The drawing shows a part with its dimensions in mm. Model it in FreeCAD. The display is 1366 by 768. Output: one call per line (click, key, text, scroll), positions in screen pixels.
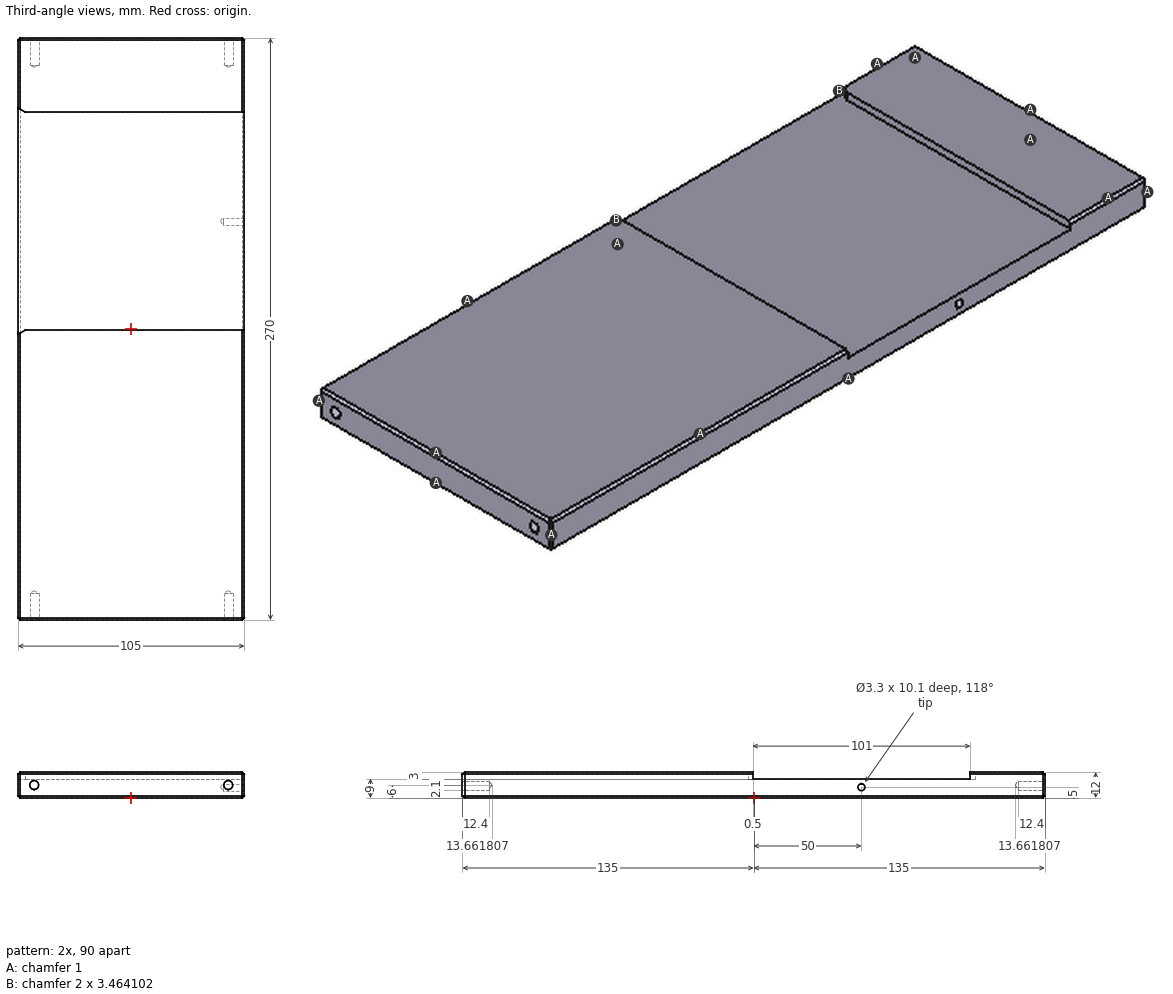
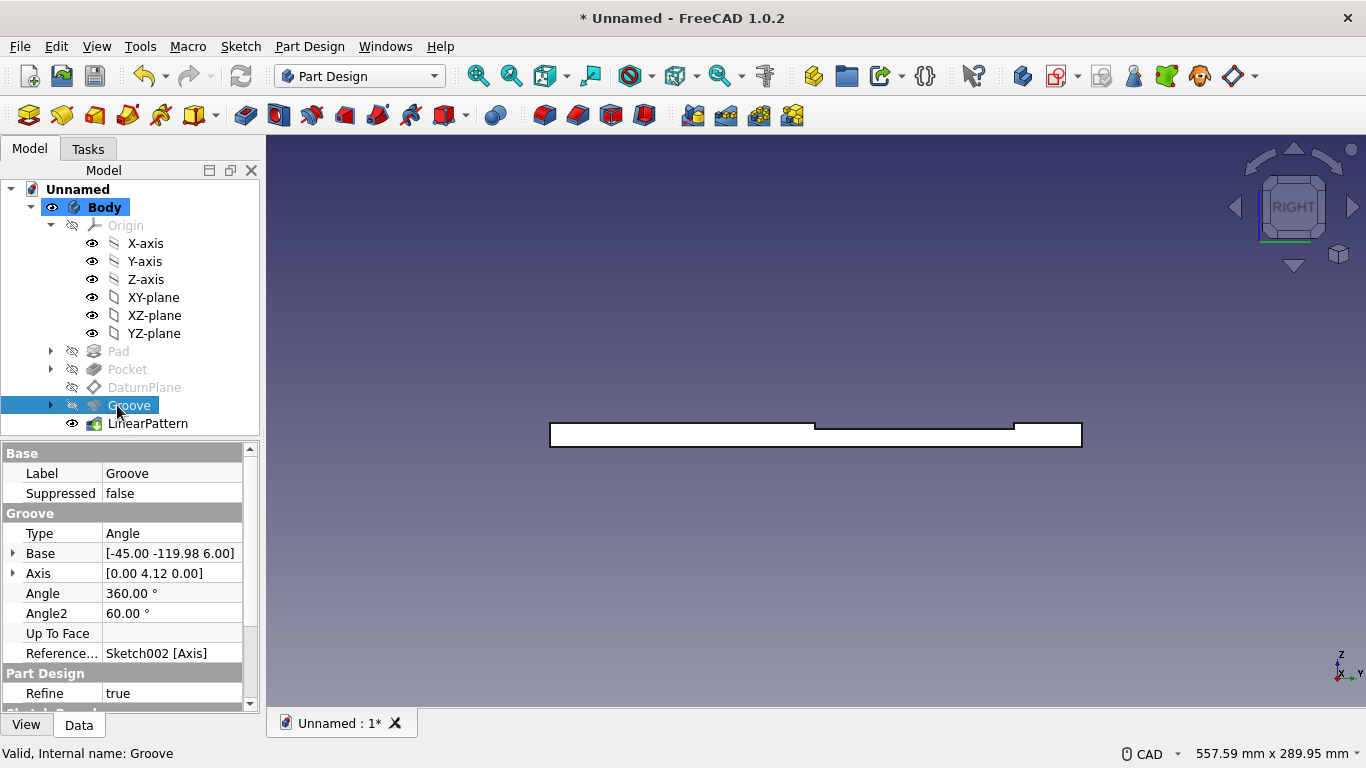
click(693, 116)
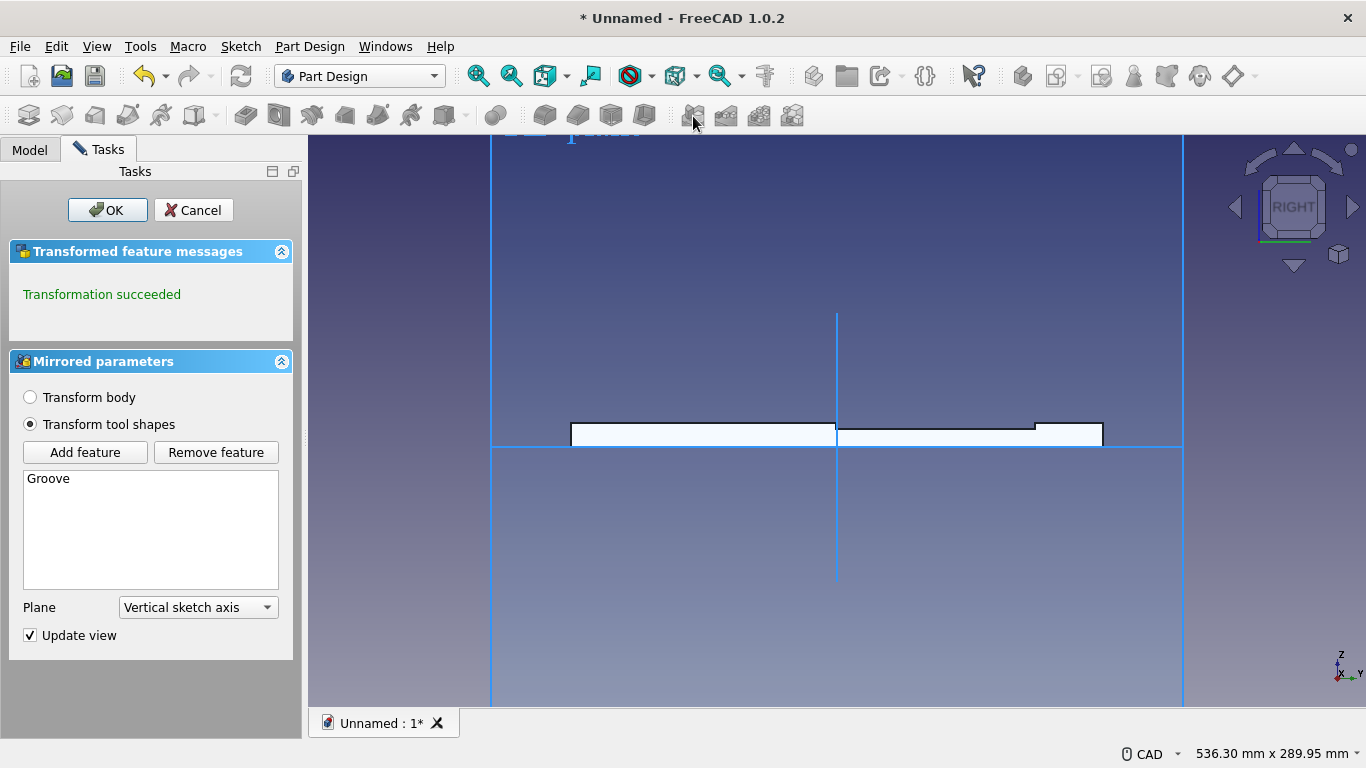
click(199, 608)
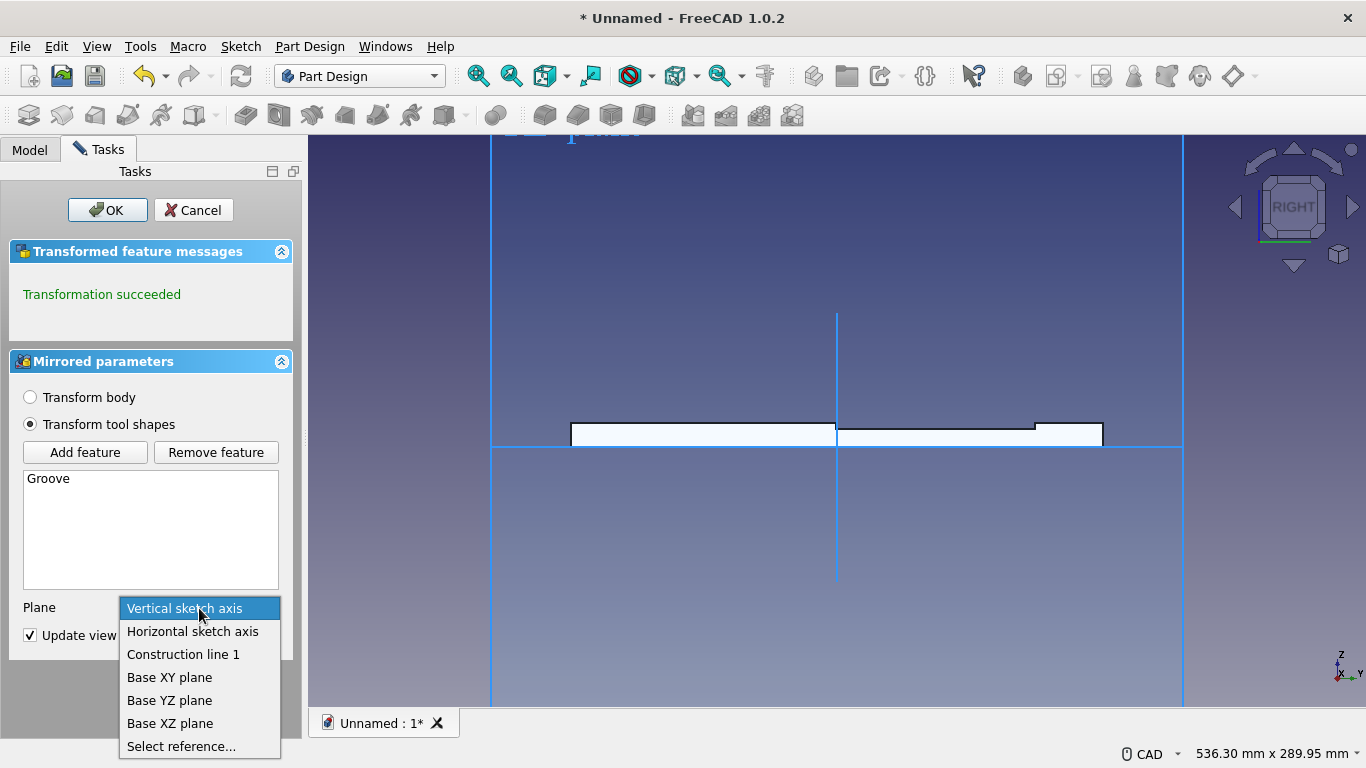
click(198, 724)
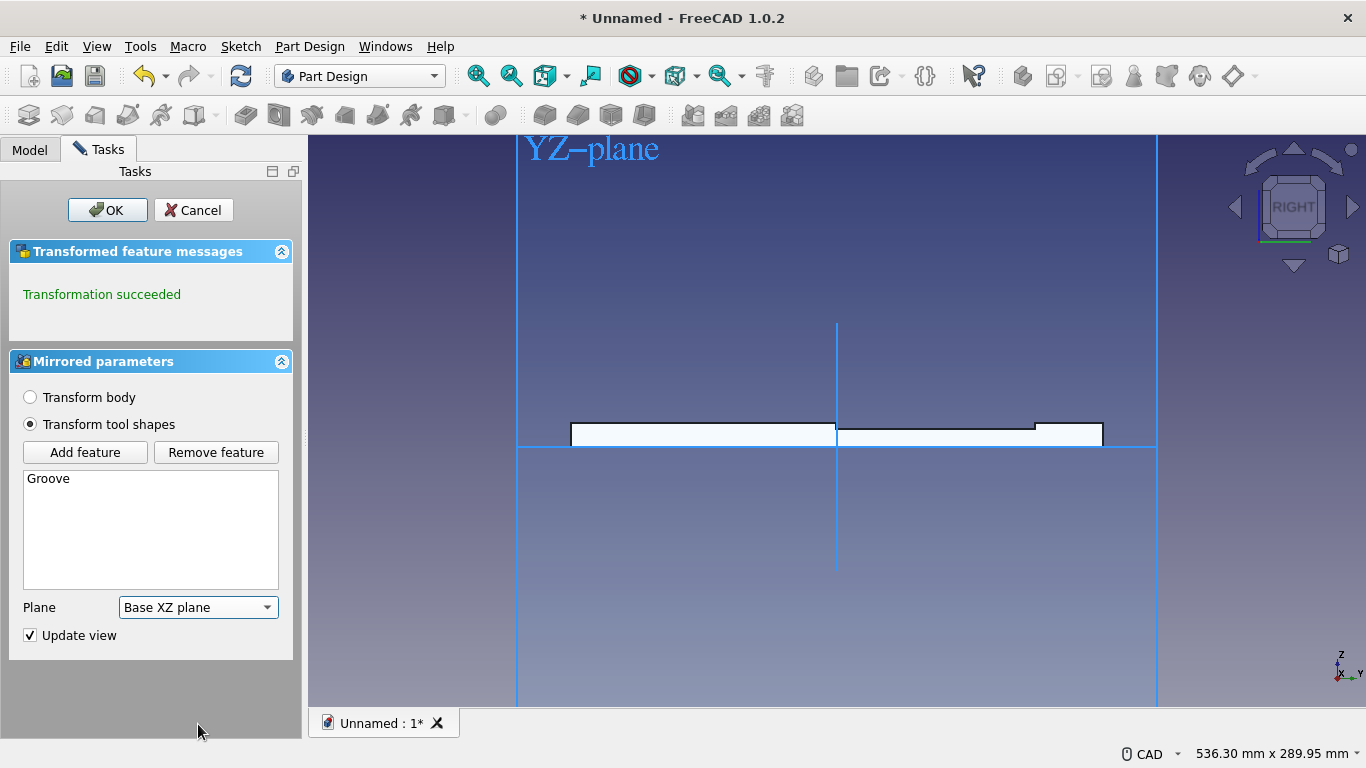
click(108, 210)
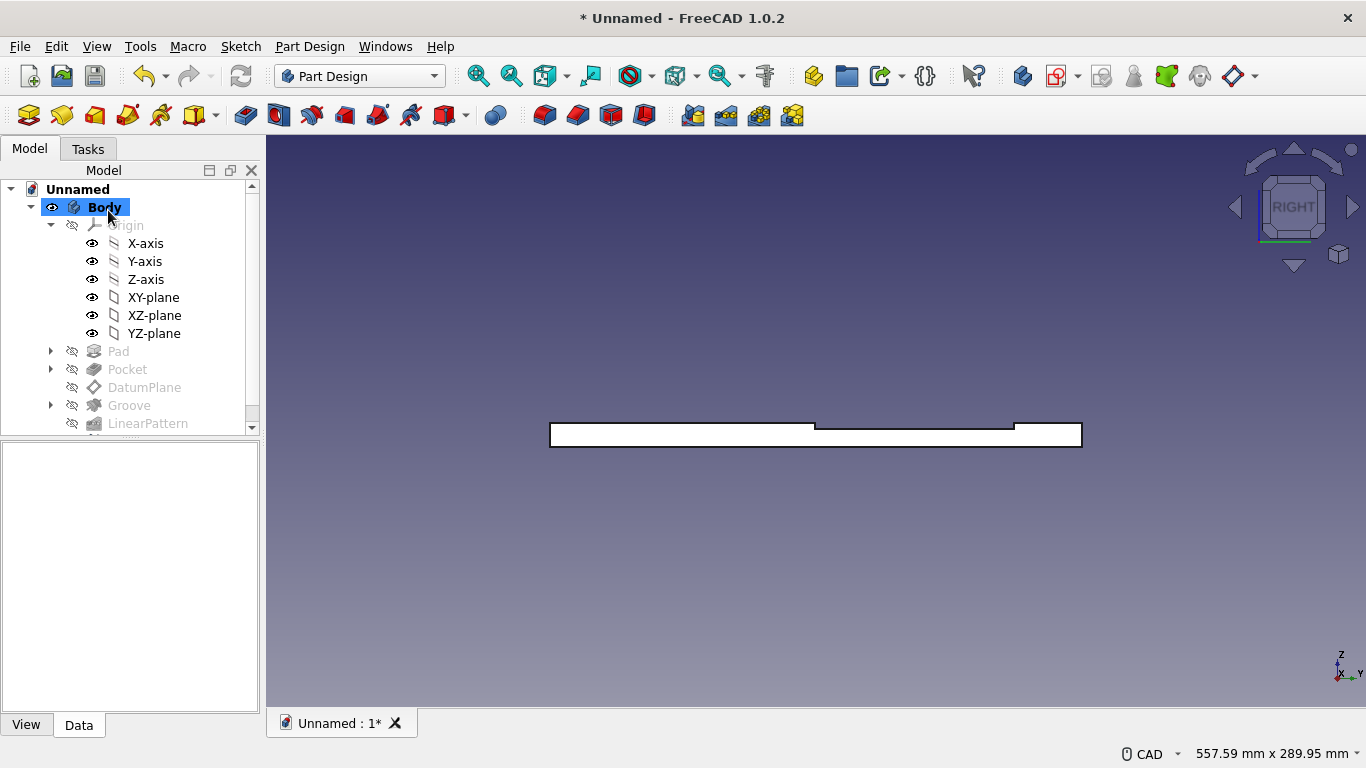
click(137, 333)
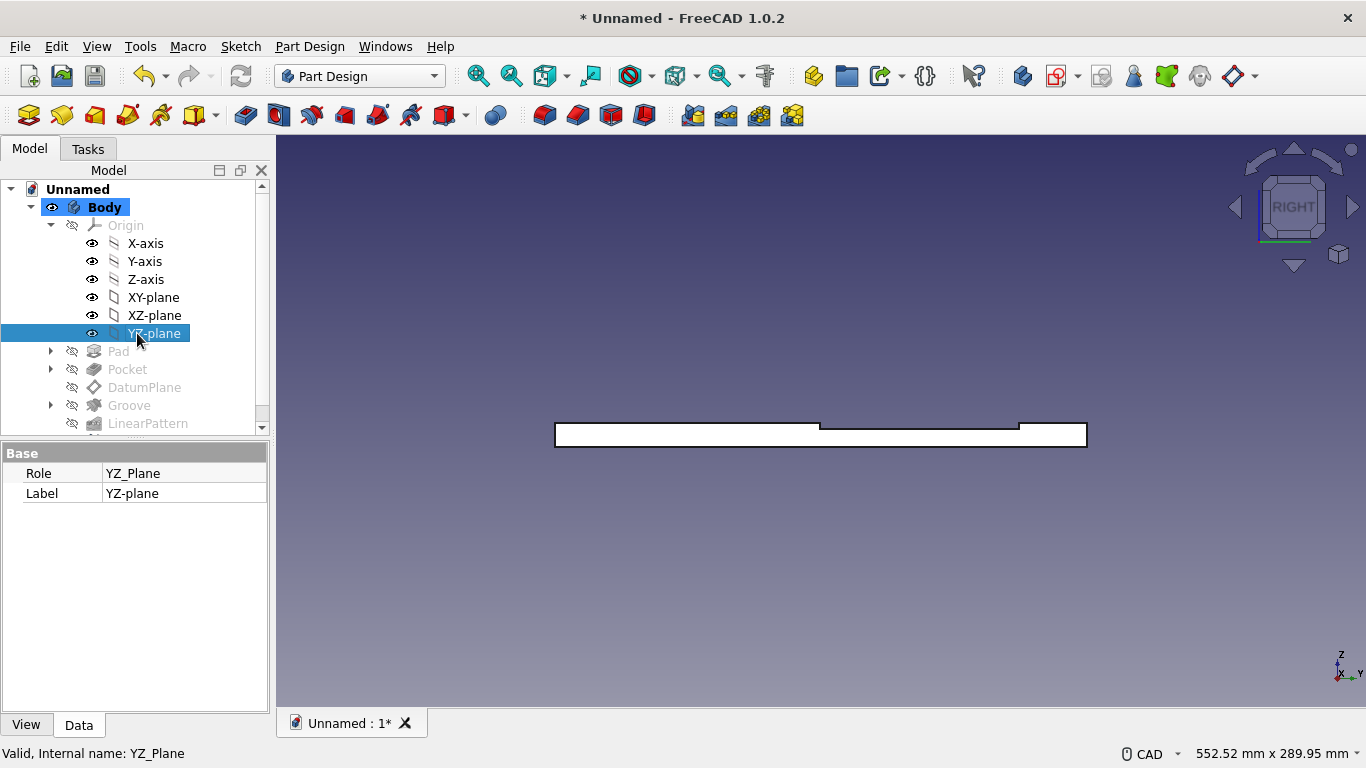
click(1232, 76)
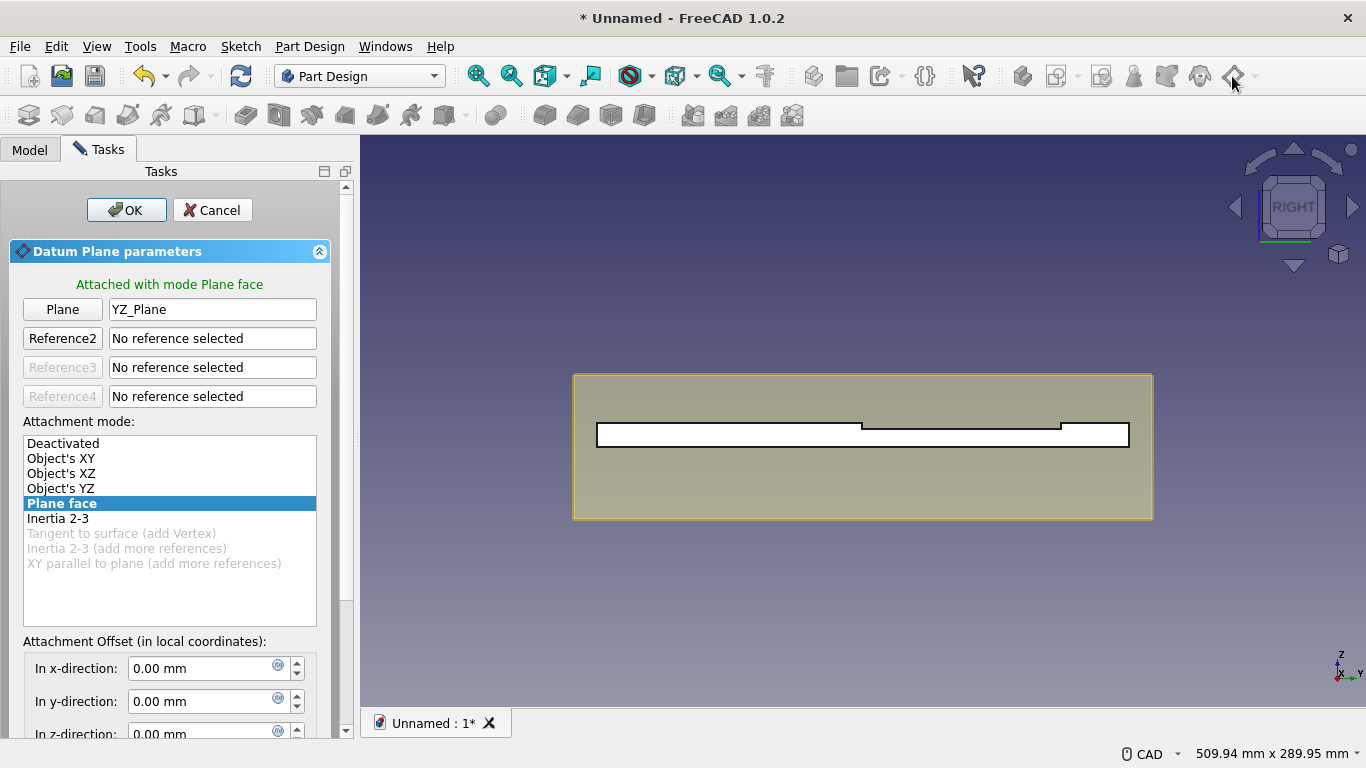
scroll(346, 460, down, 2)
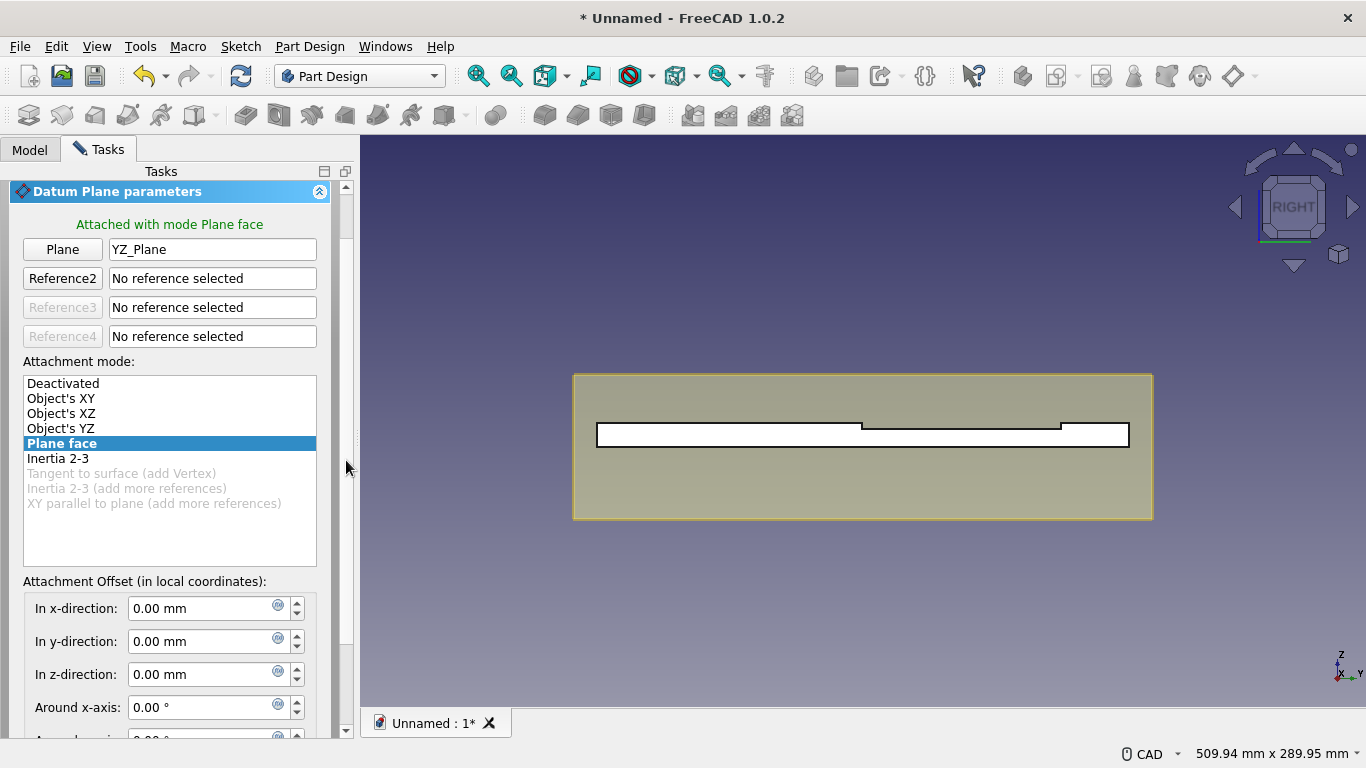
triple_click(210, 614)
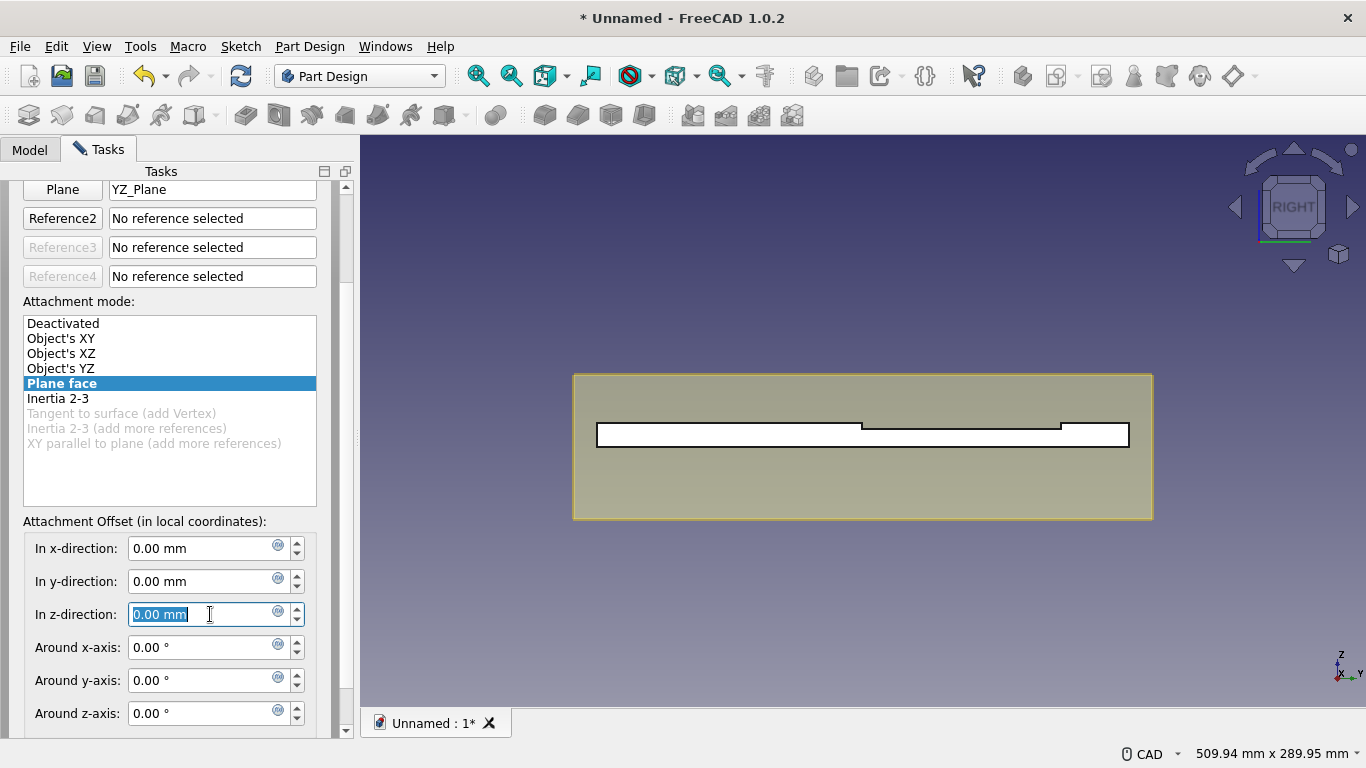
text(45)
key(Tab)